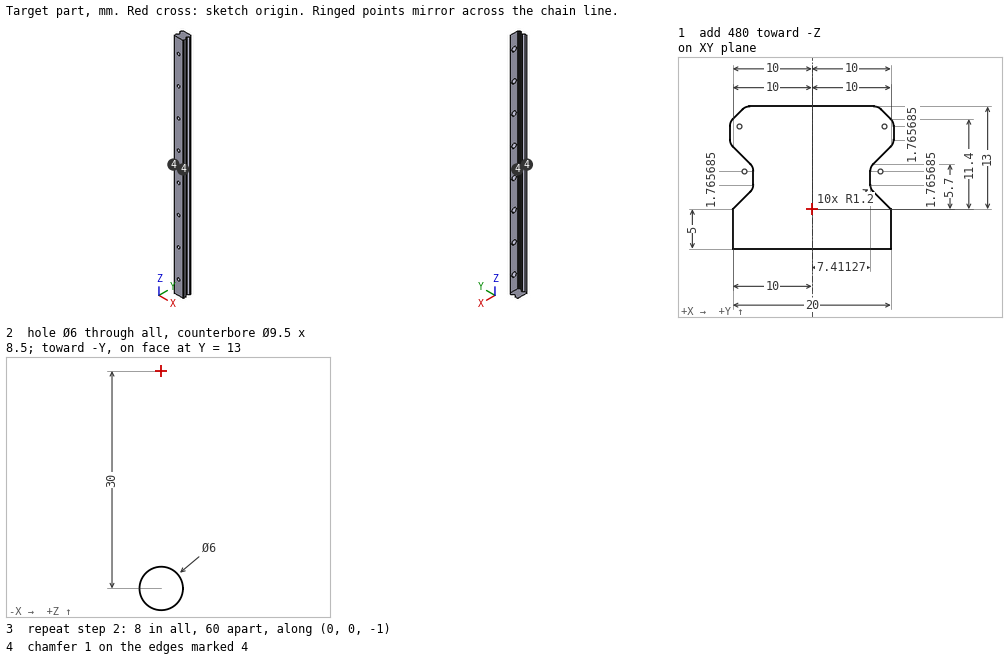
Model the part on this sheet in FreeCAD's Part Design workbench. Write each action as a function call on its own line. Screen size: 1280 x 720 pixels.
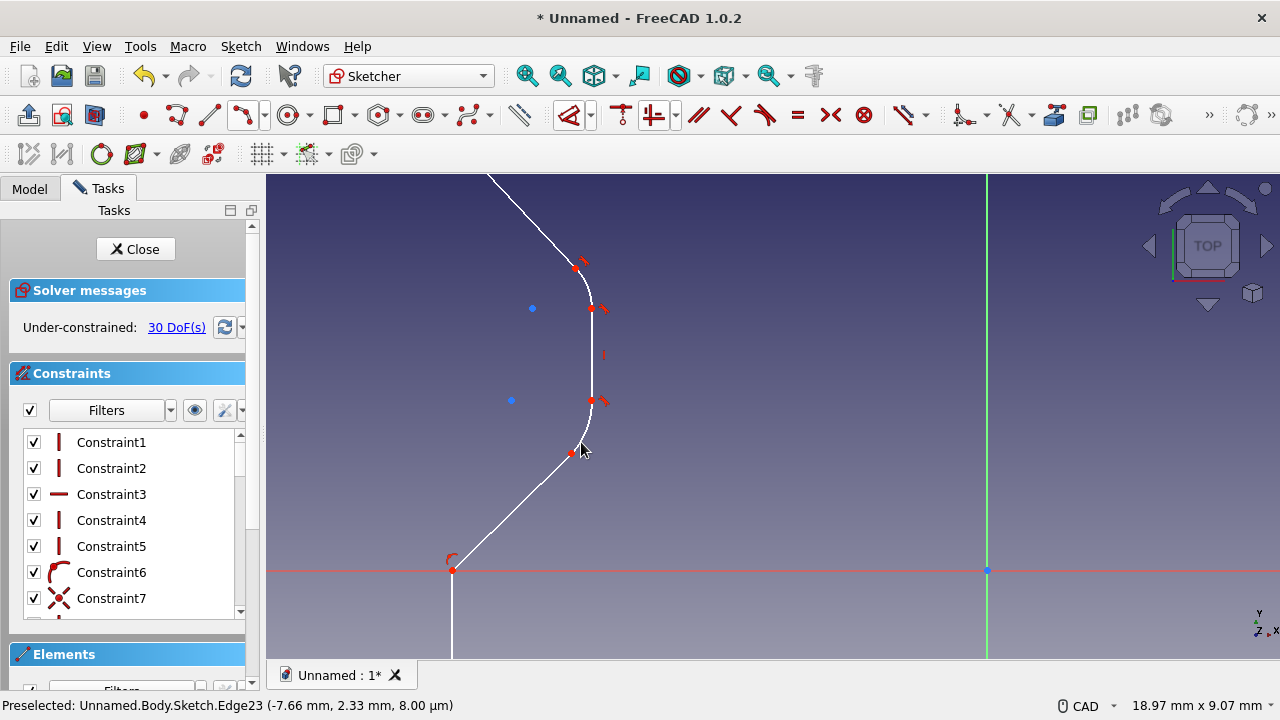
click(536, 489)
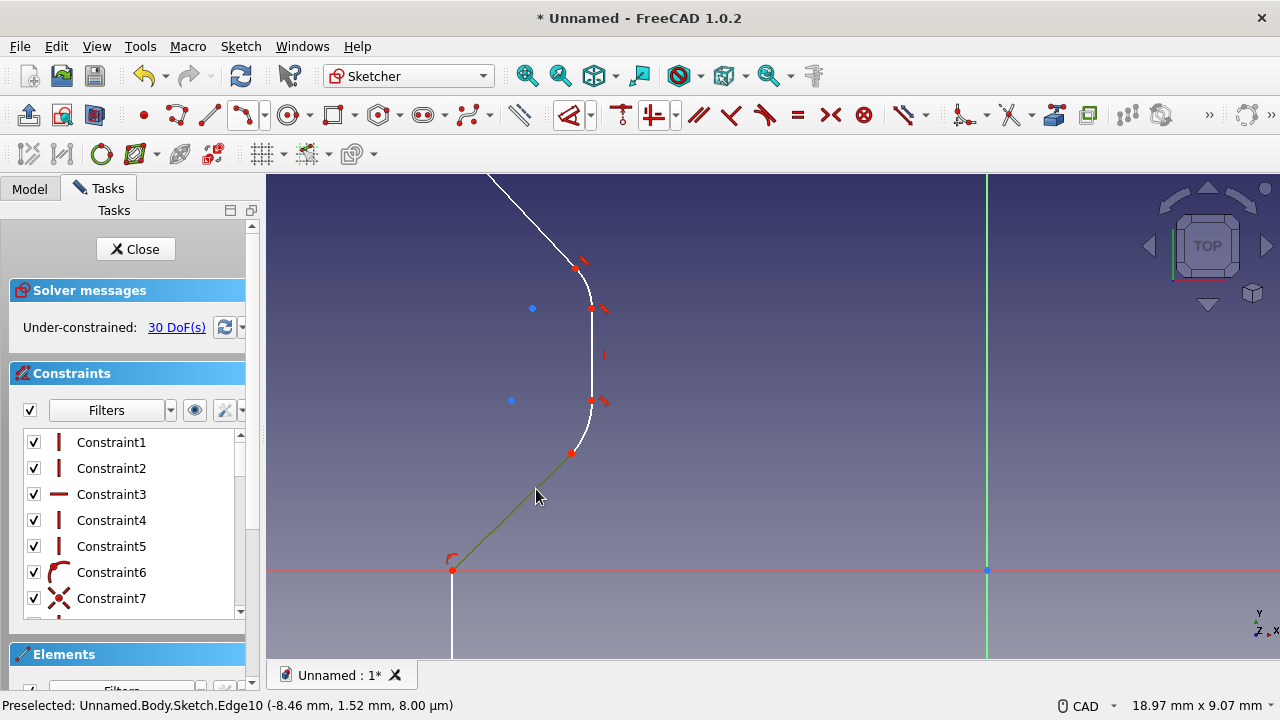
click(582, 440)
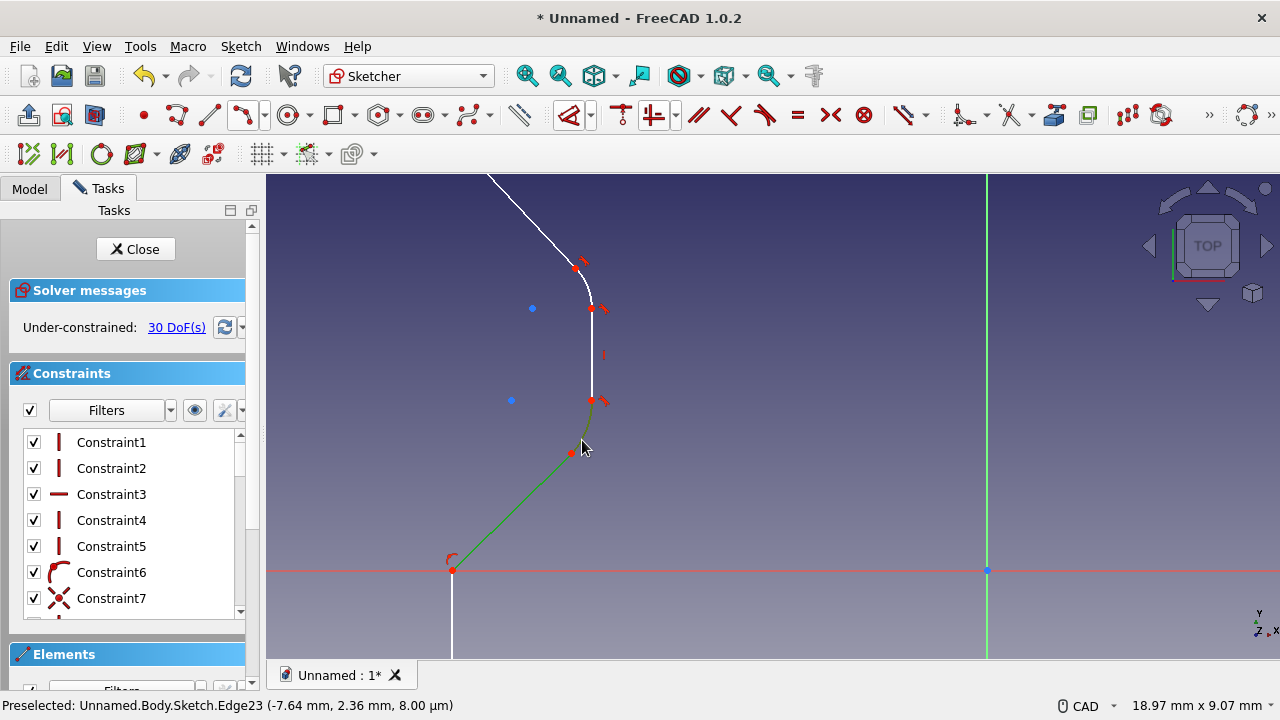
key(t)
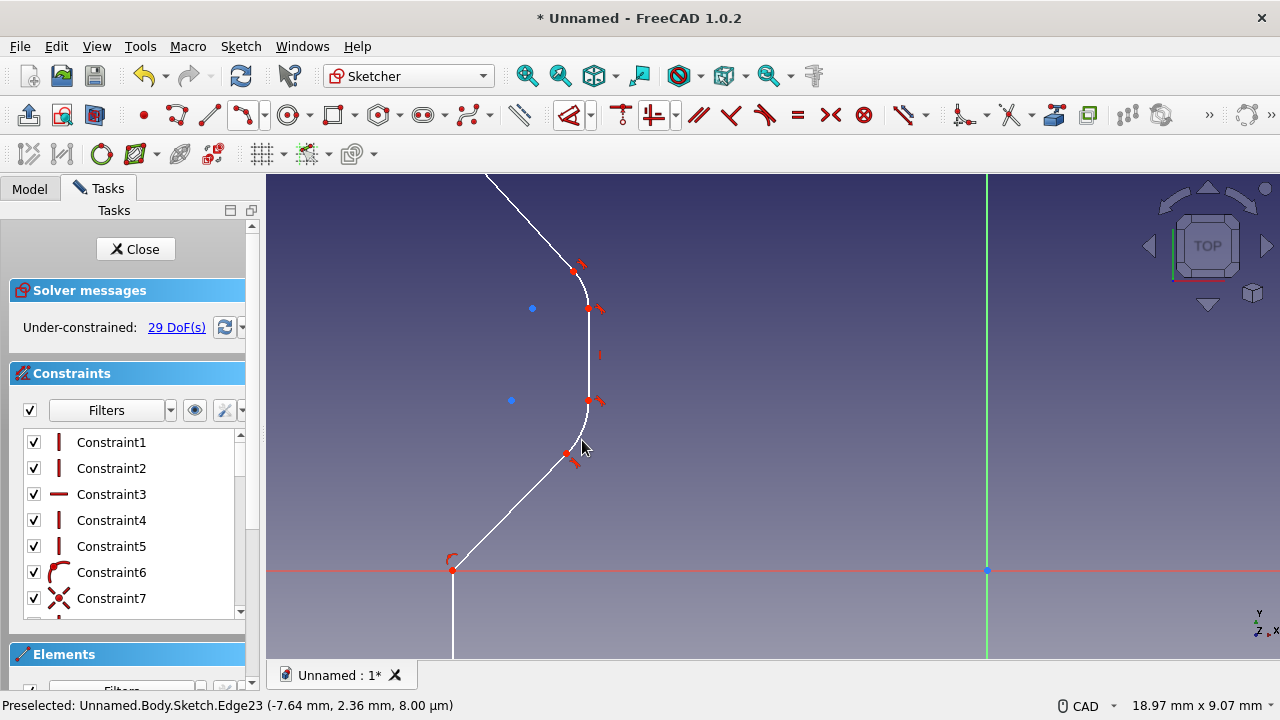
scroll(583, 442, down, 6)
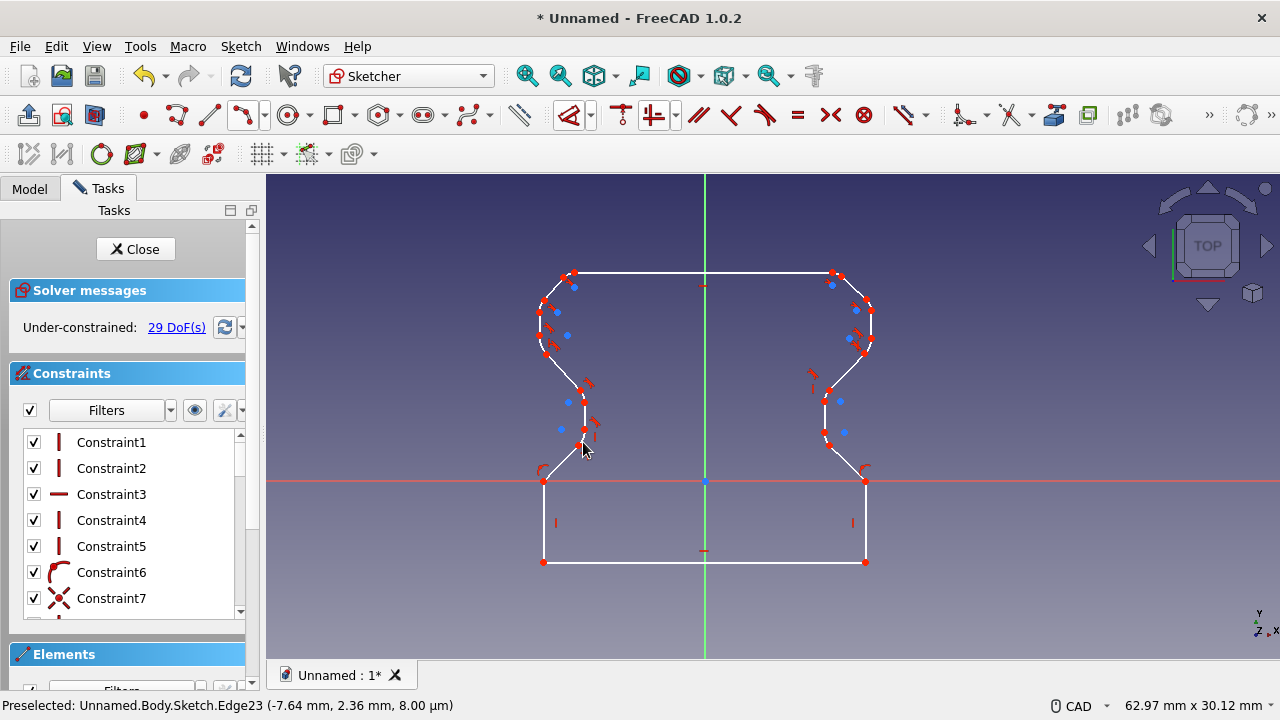
scroll(855, 471, up, 2)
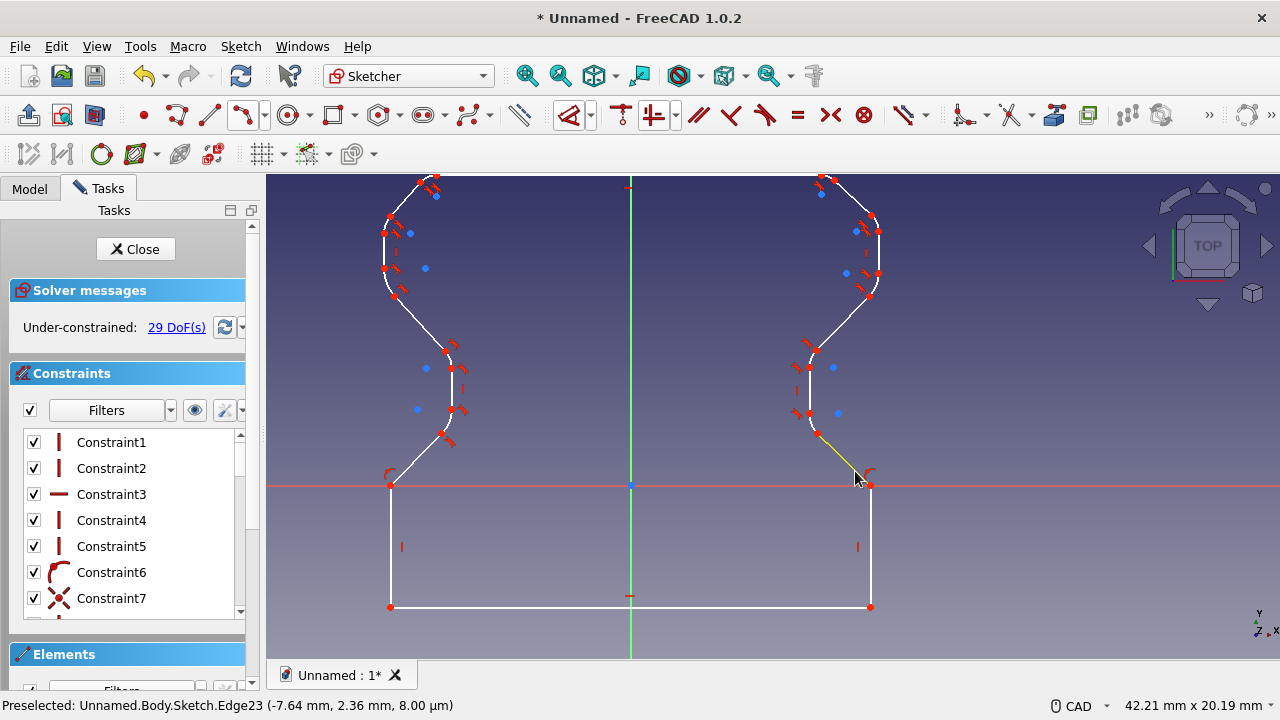
click(855, 470)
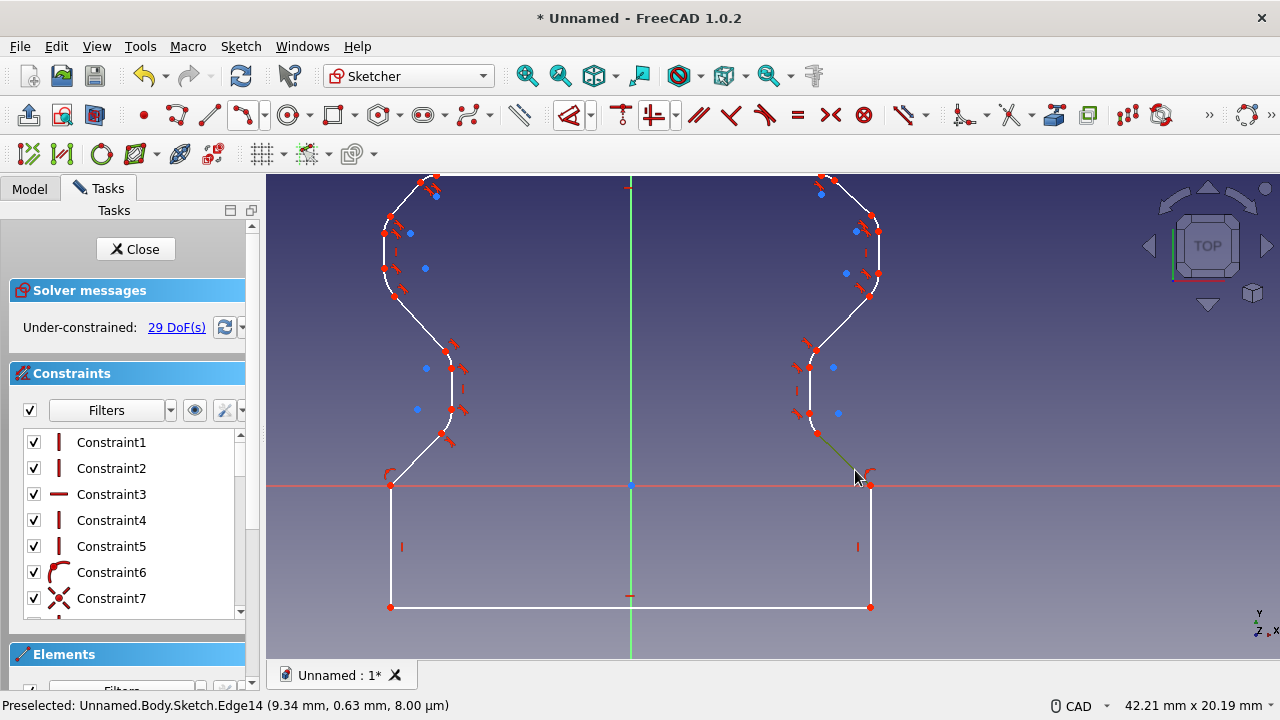
scroll(812, 424, up, 2)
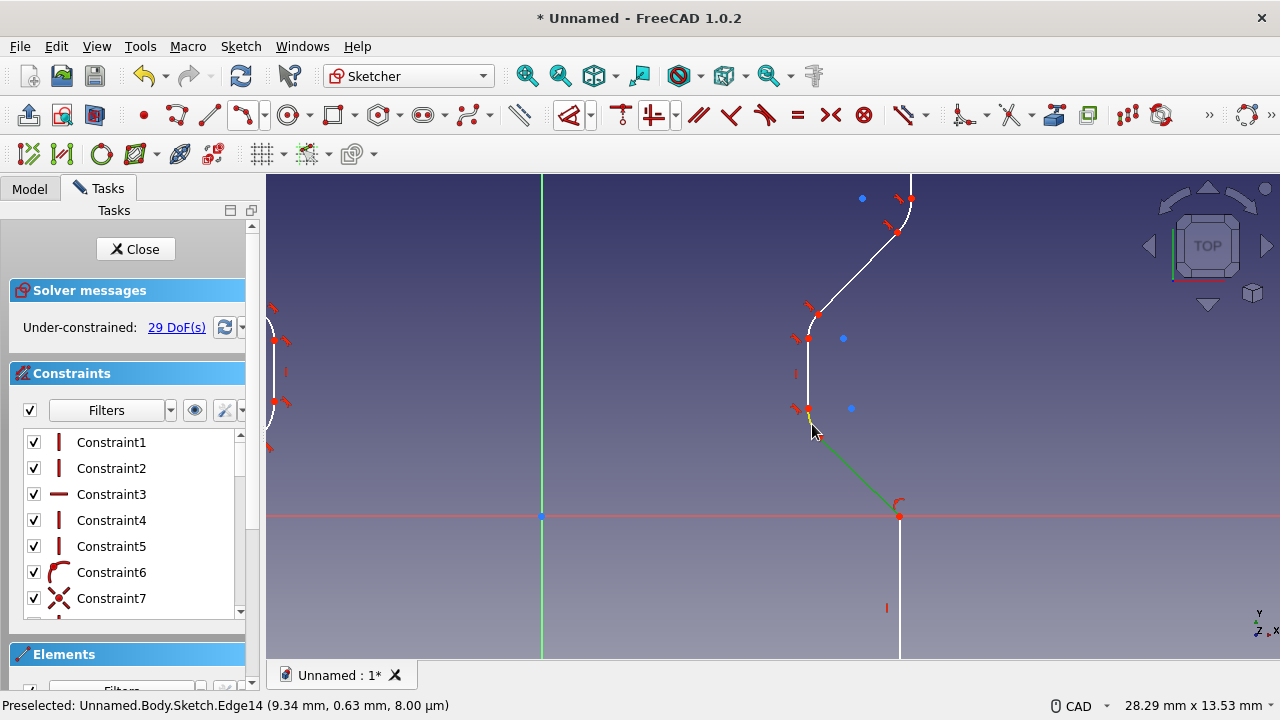
click(811, 424)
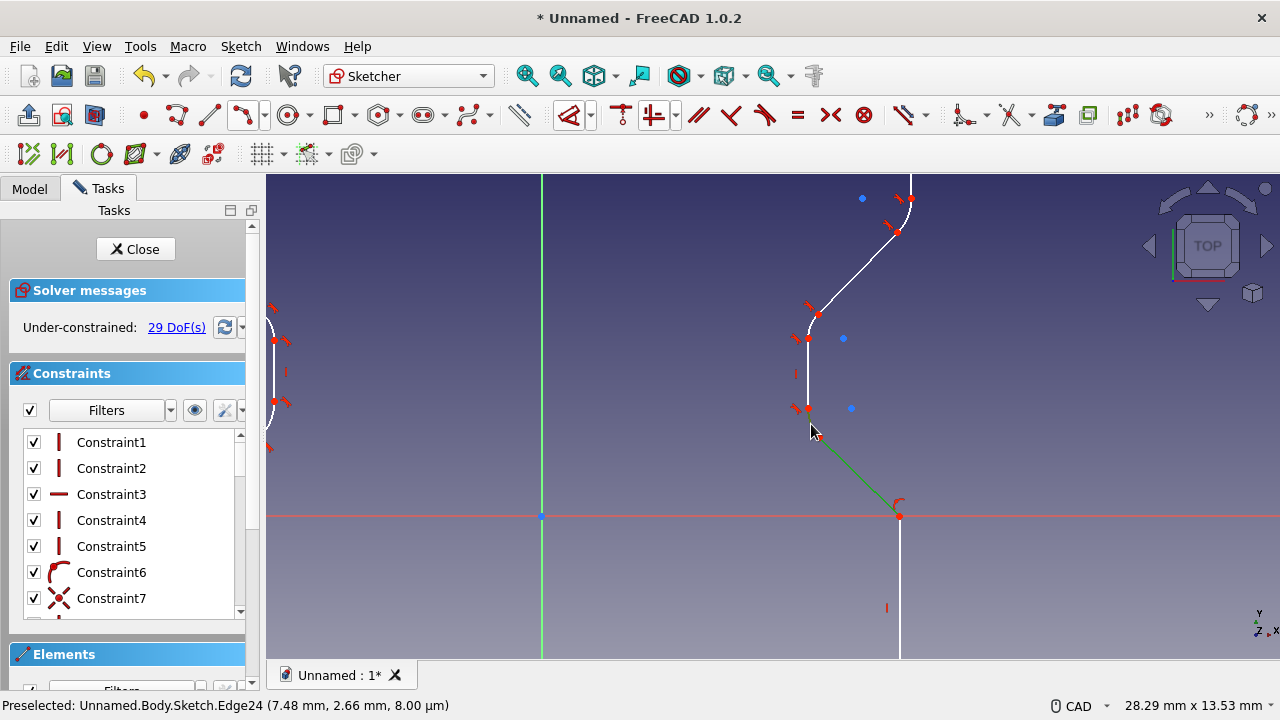
key(t)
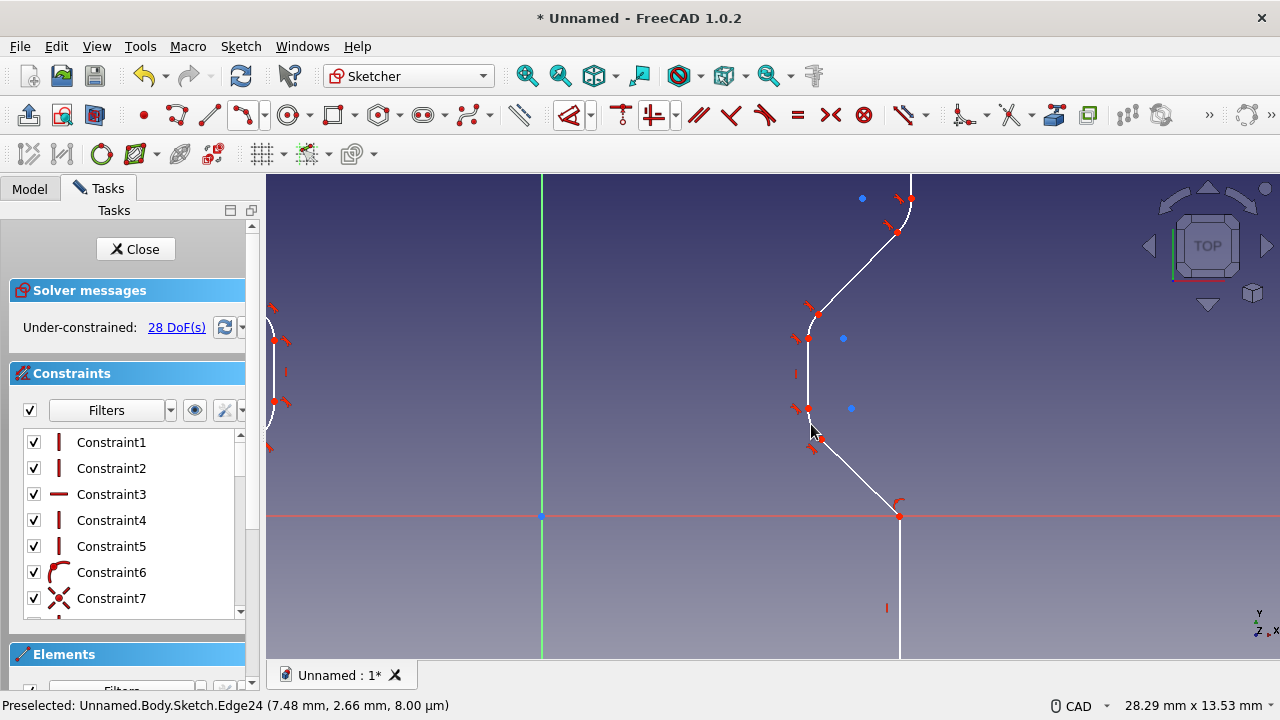
click(811, 326)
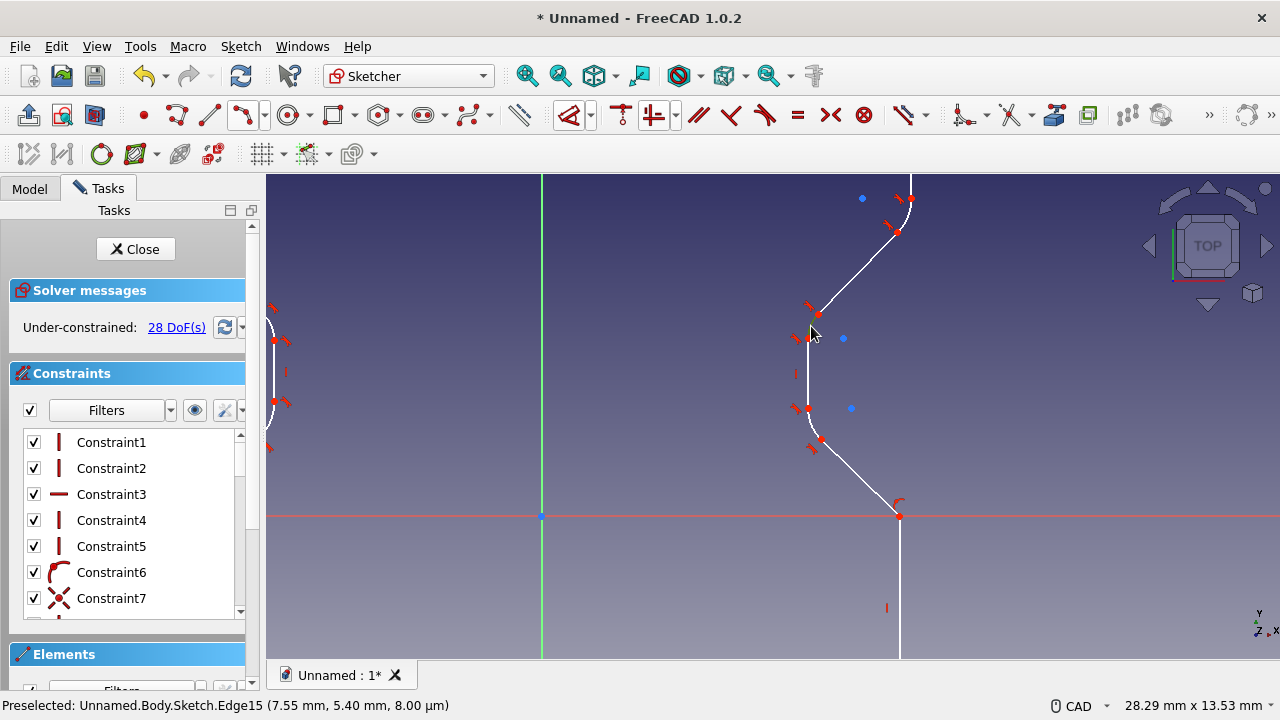
scroll(904, 224, up, 2)